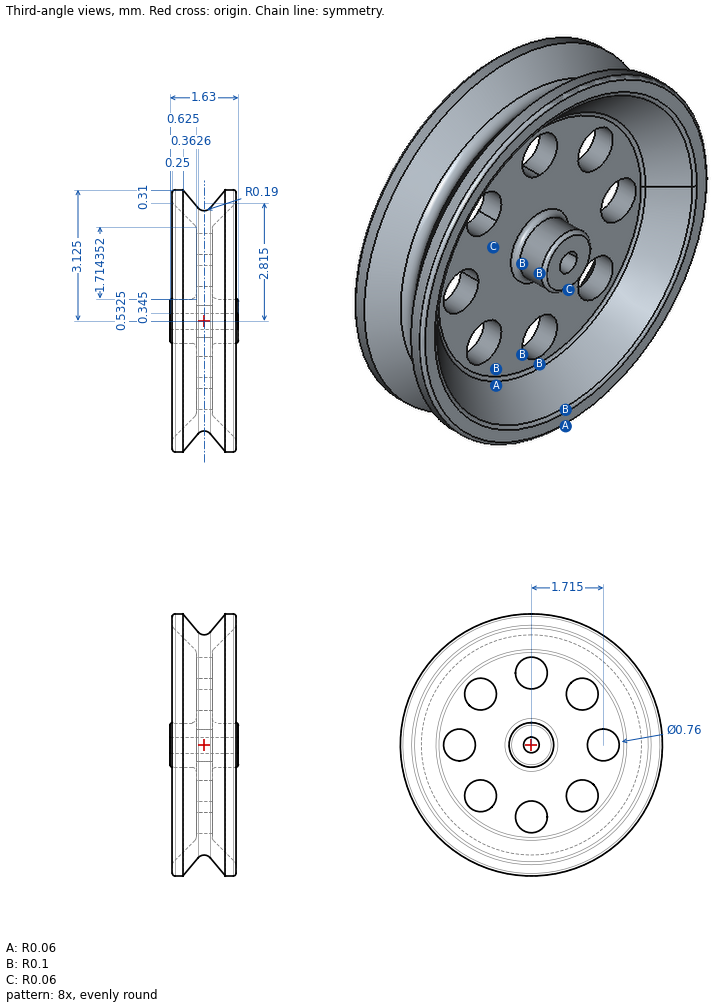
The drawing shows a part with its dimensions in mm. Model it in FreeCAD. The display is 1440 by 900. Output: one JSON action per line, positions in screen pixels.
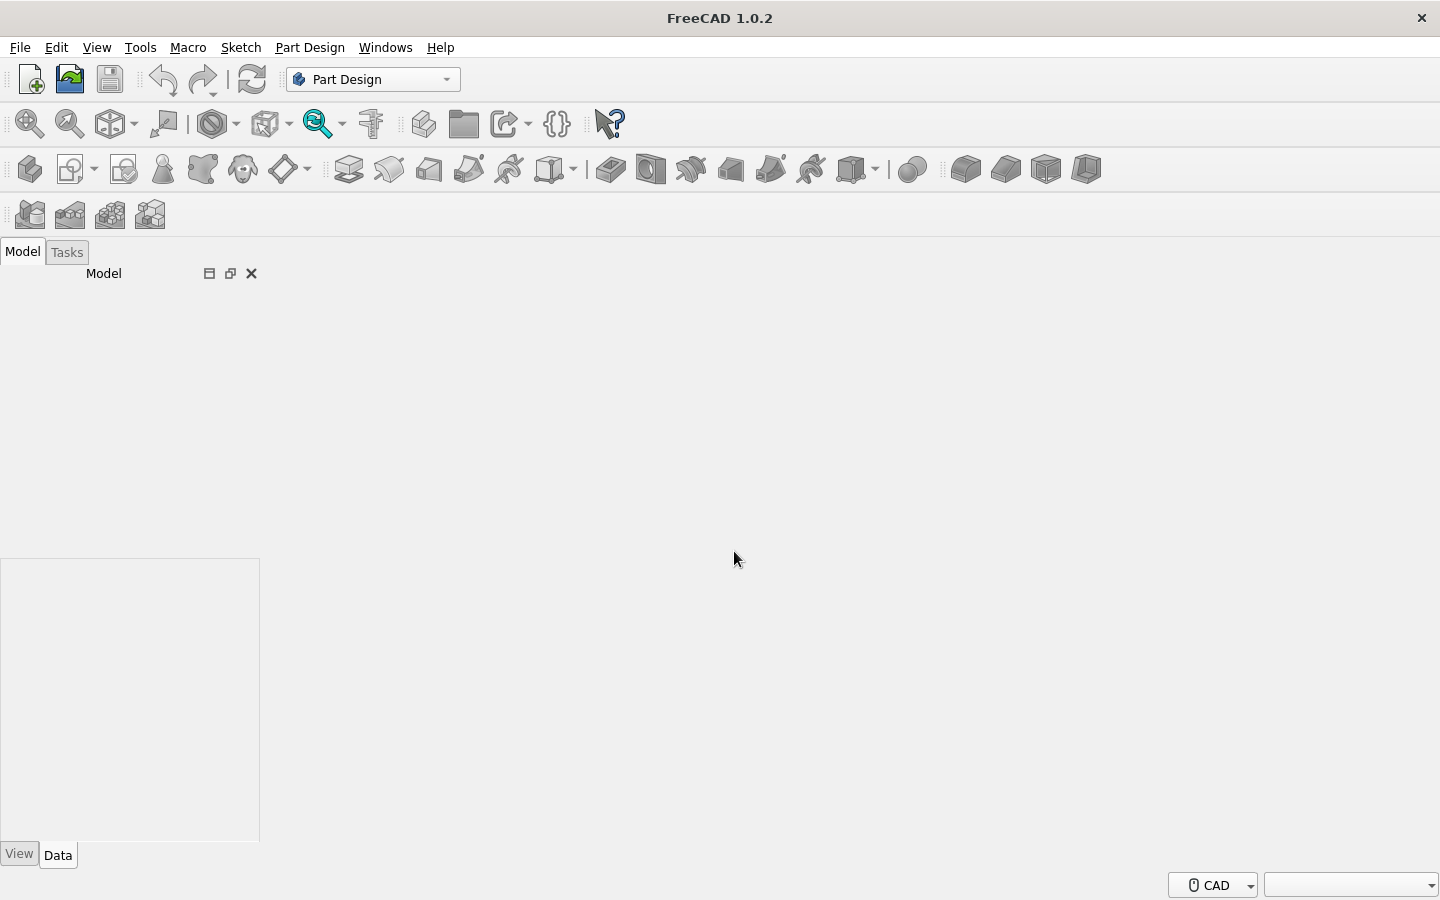
{"action": "left_click", "coordinate": [30, 80]}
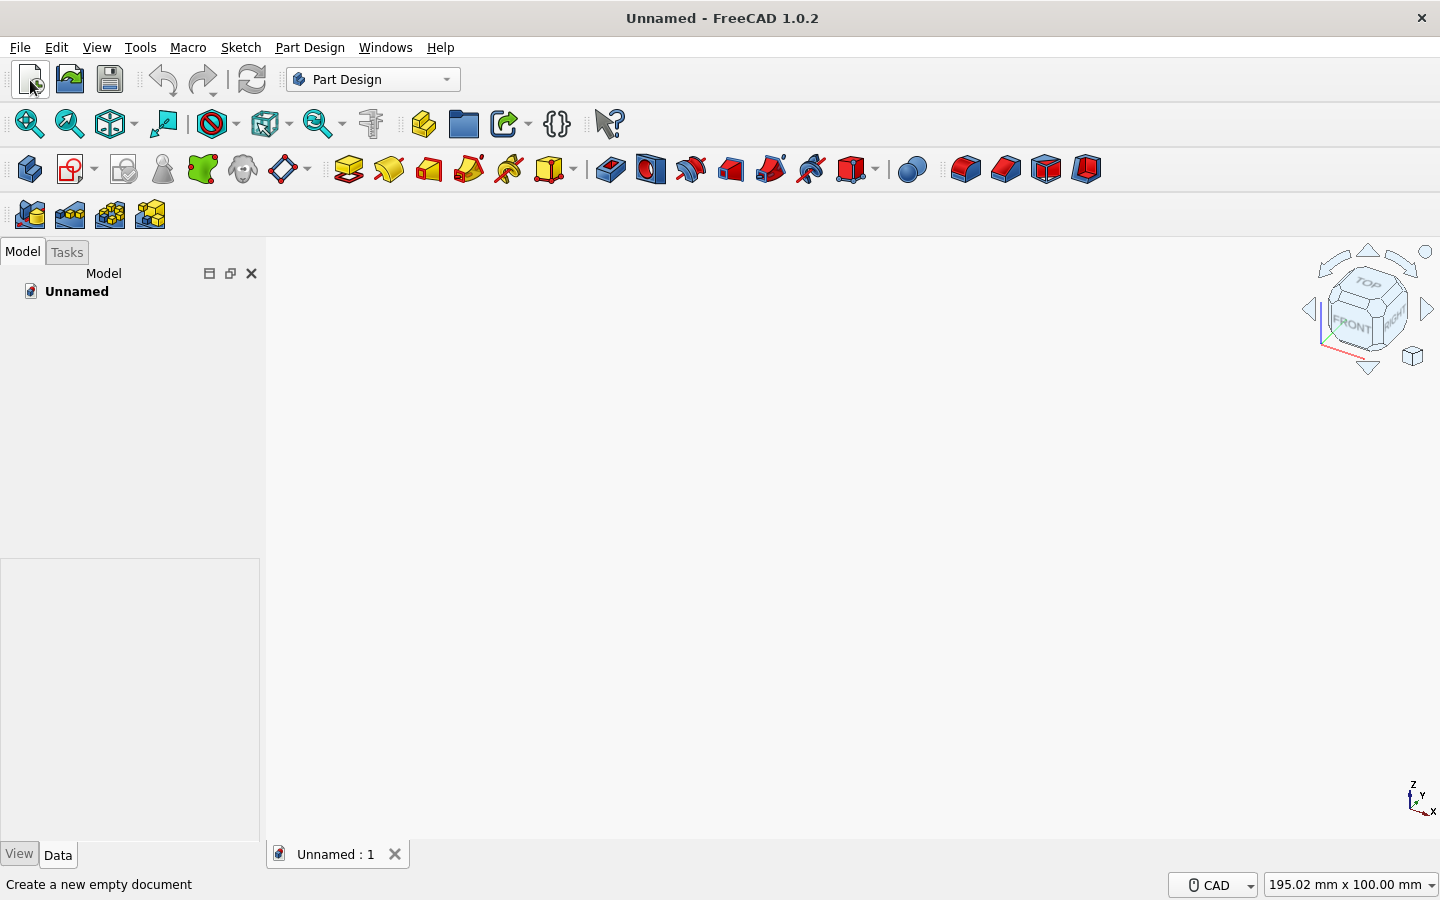
{"action": "left_click", "coordinate": [70, 170]}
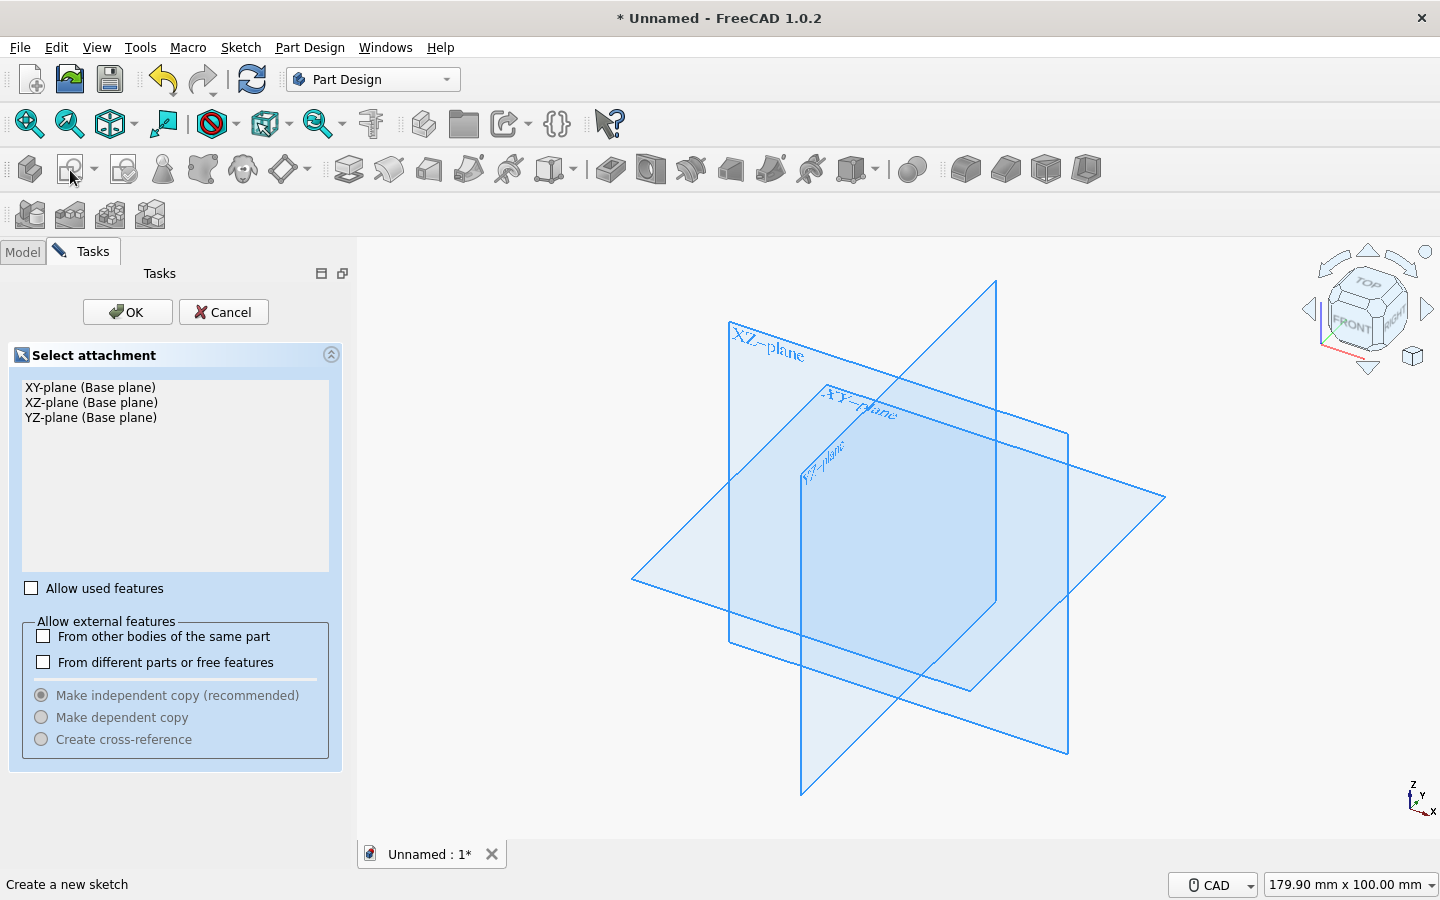
{"action": "left_click", "coordinate": [82, 388]}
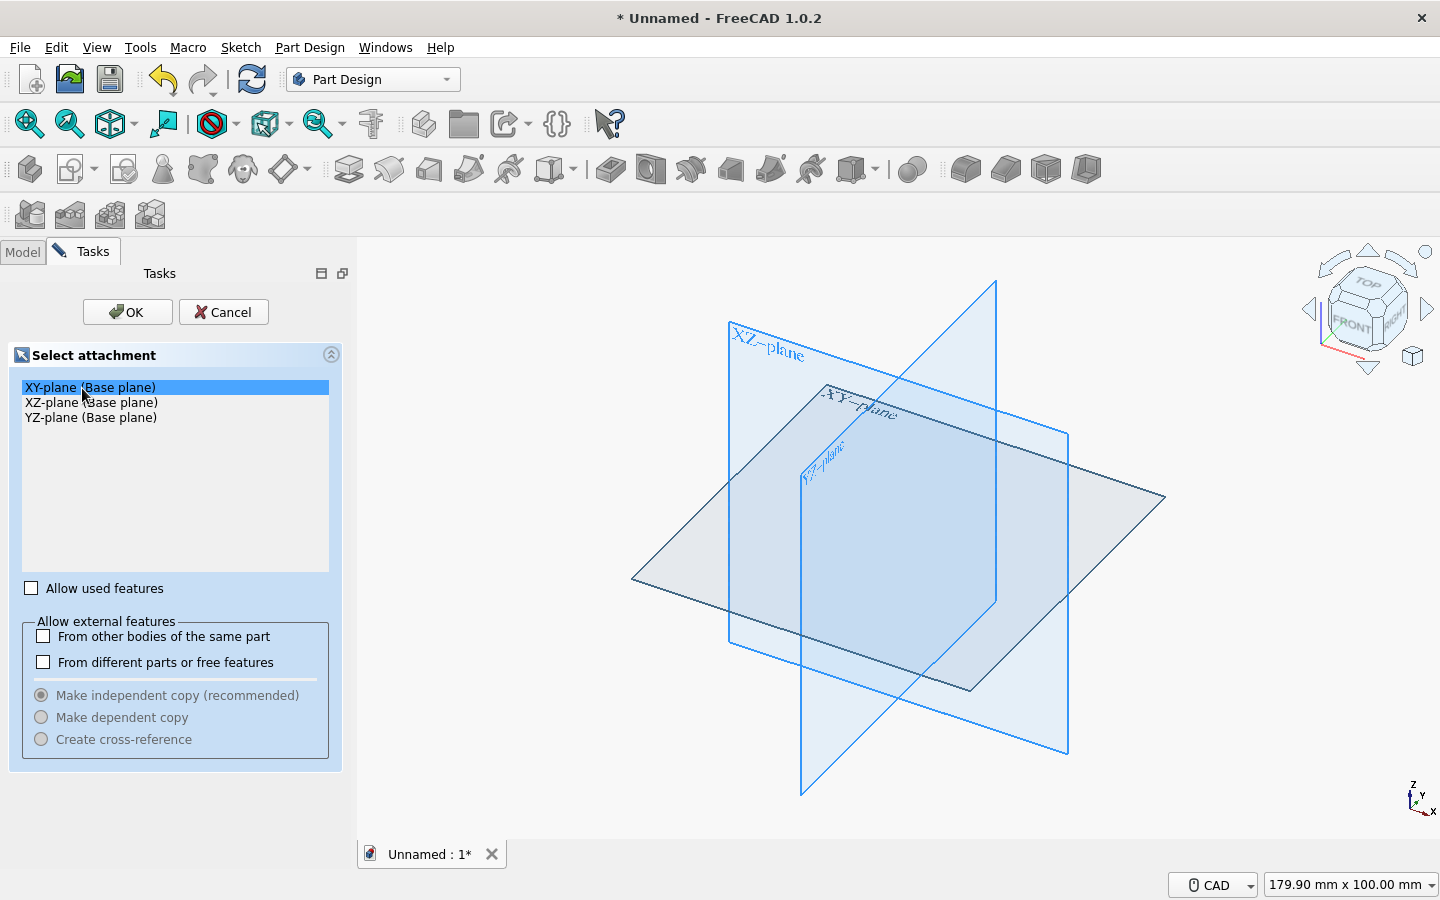
{"action": "left_click", "coordinate": [128, 312]}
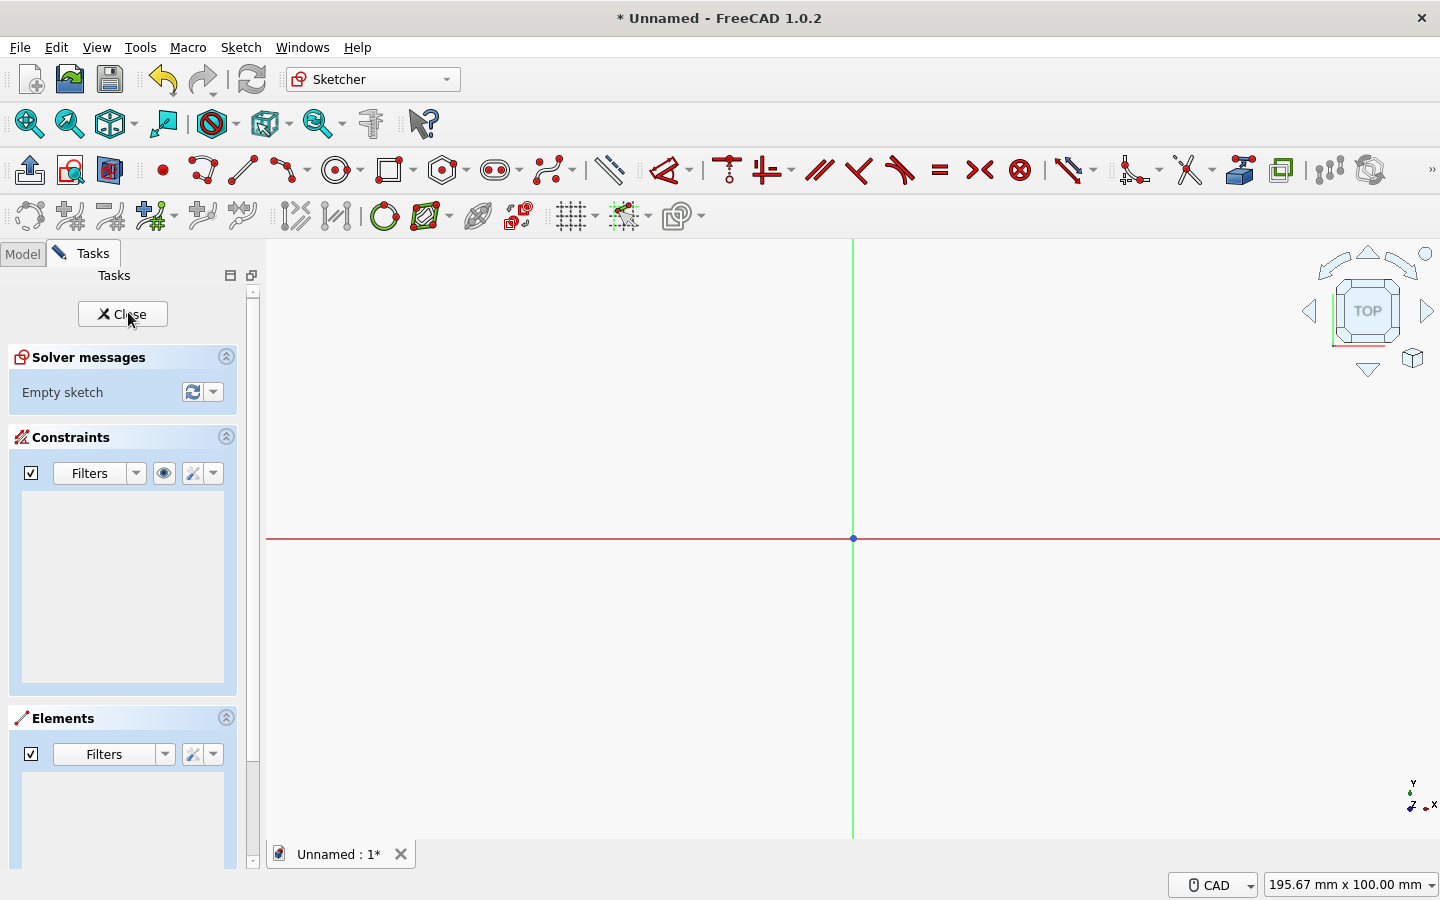
{"action": "scroll", "coordinate": [857, 529], "scroll_direction": "up", "scroll_amount": 15}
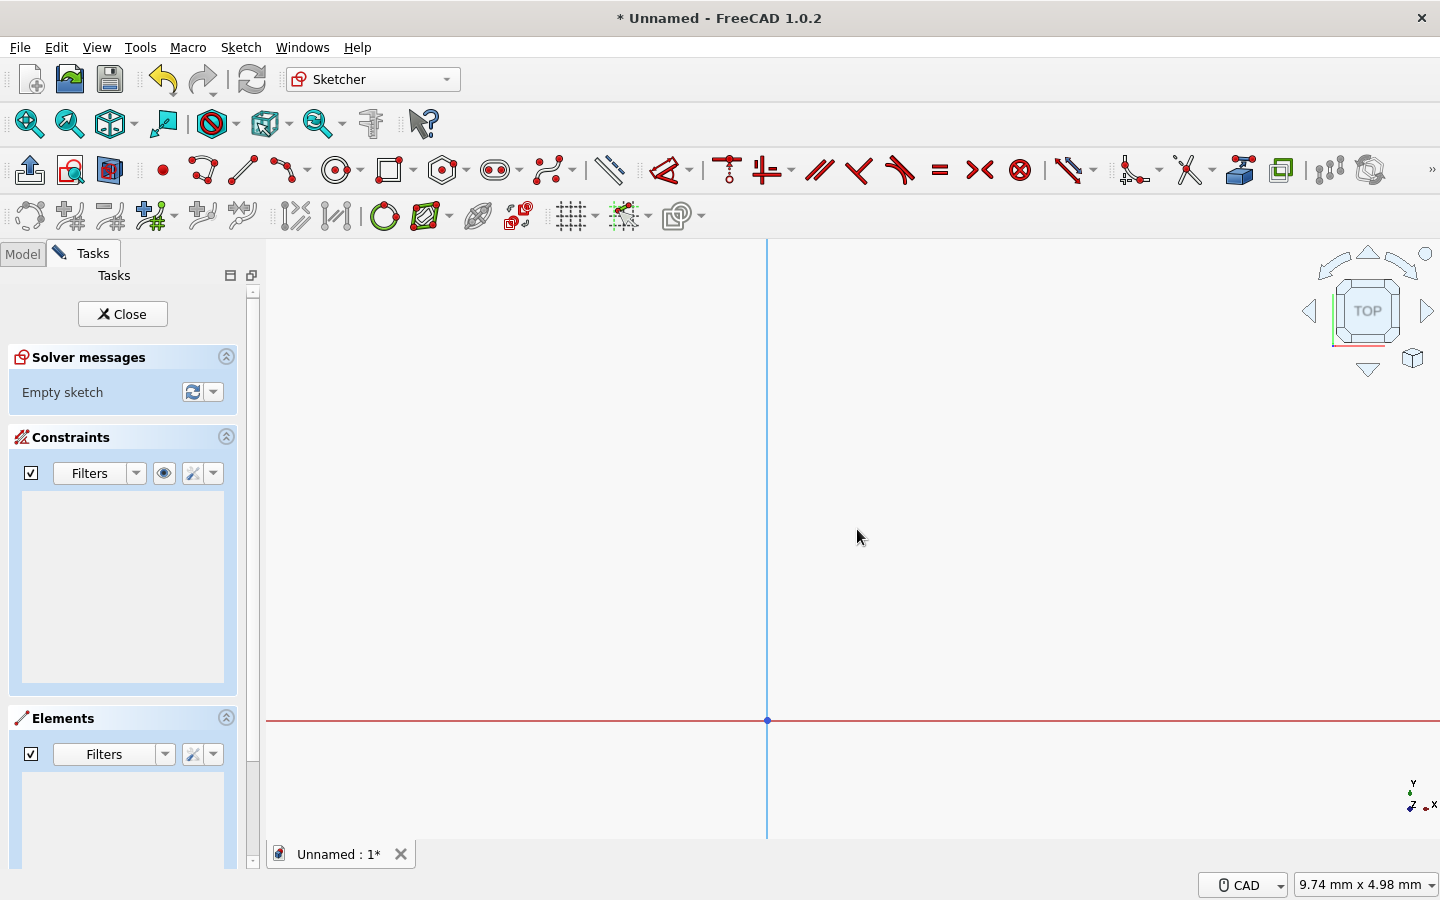
{"action": "left_click", "coordinate": [204, 170]}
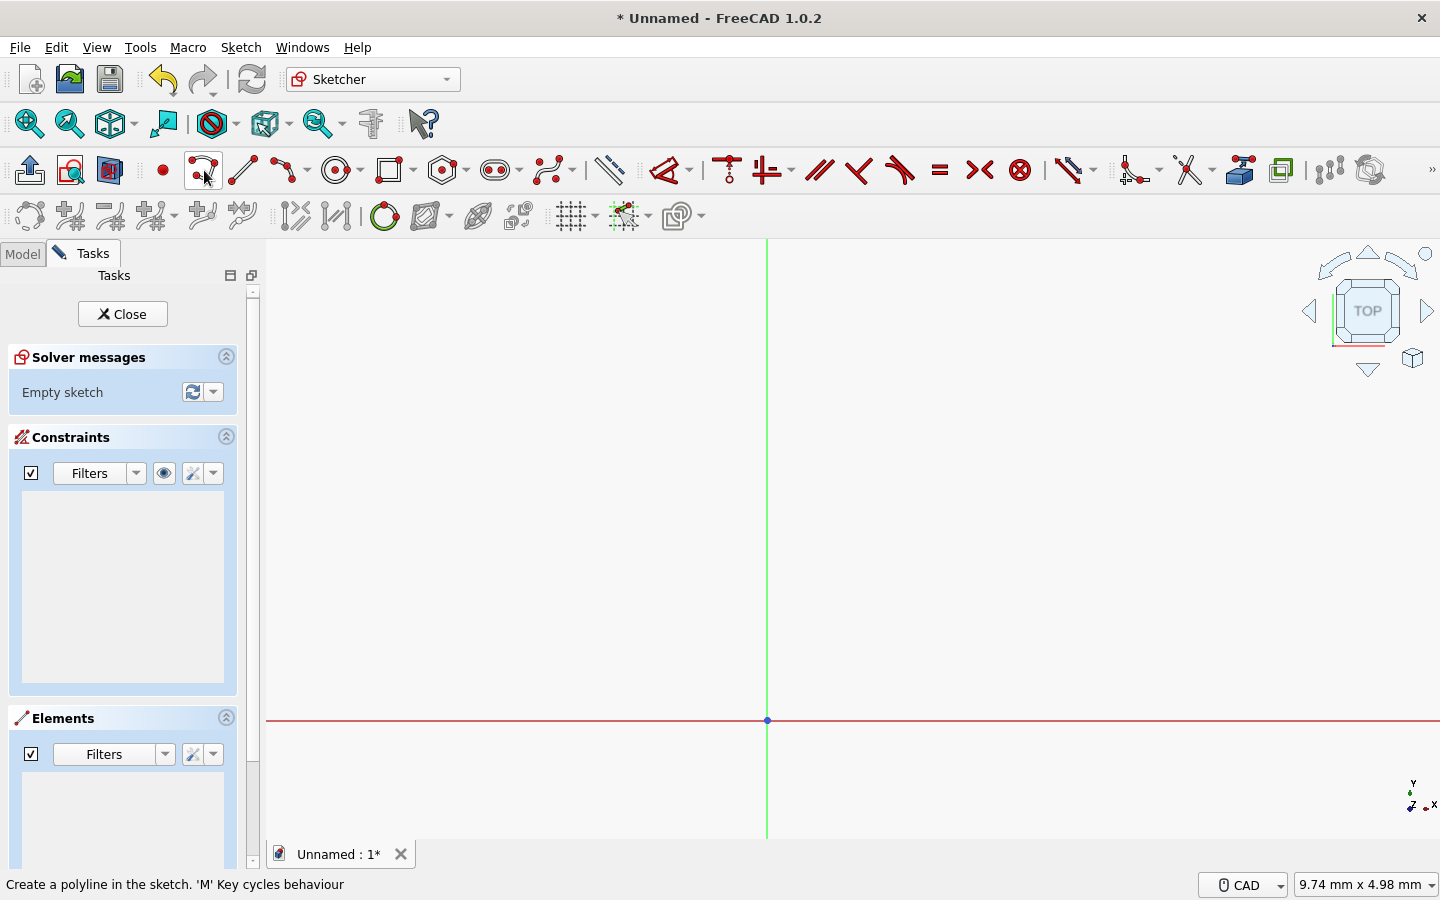
{"action": "left_click", "coordinate": [750, 396]}
{"action": "left_click", "coordinate": [706, 344]}
{"action": "left_click", "coordinate": [676, 344]}
{"action": "left_click", "coordinate": [676, 381]}
{"action": "left_click", "coordinate": [744, 450]}
{"action": "left_click", "coordinate": [744, 656]}
{"action": "left_click", "coordinate": [669, 656]}
{"action": "left_click", "coordinate": [669, 698]}
{"action": "left_click", "coordinate": [865, 698]}
{"action": "left_click", "coordinate": [865, 656]}
{"action": "left_click", "coordinate": [790, 656]}
{"action": "left_click", "coordinate": [790, 450]}
{"action": "left_click", "coordinate": [858, 381]}
{"action": "left_click", "coordinate": [858, 344]}
{"action": "left_click", "coordinate": [828, 344]}
{"action": "left_click", "coordinate": [785, 396]}
{"action": "right_click", "coordinate": [785, 396]}